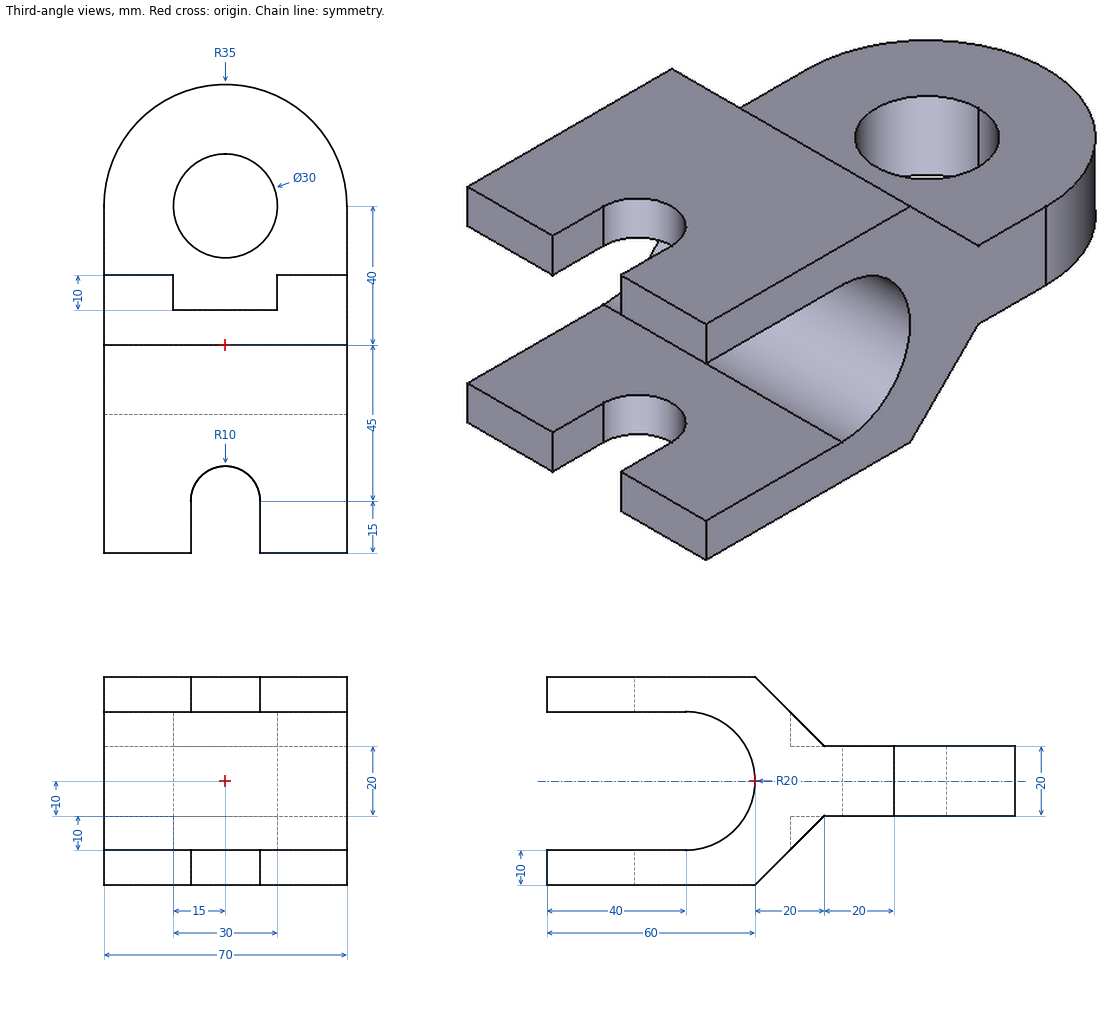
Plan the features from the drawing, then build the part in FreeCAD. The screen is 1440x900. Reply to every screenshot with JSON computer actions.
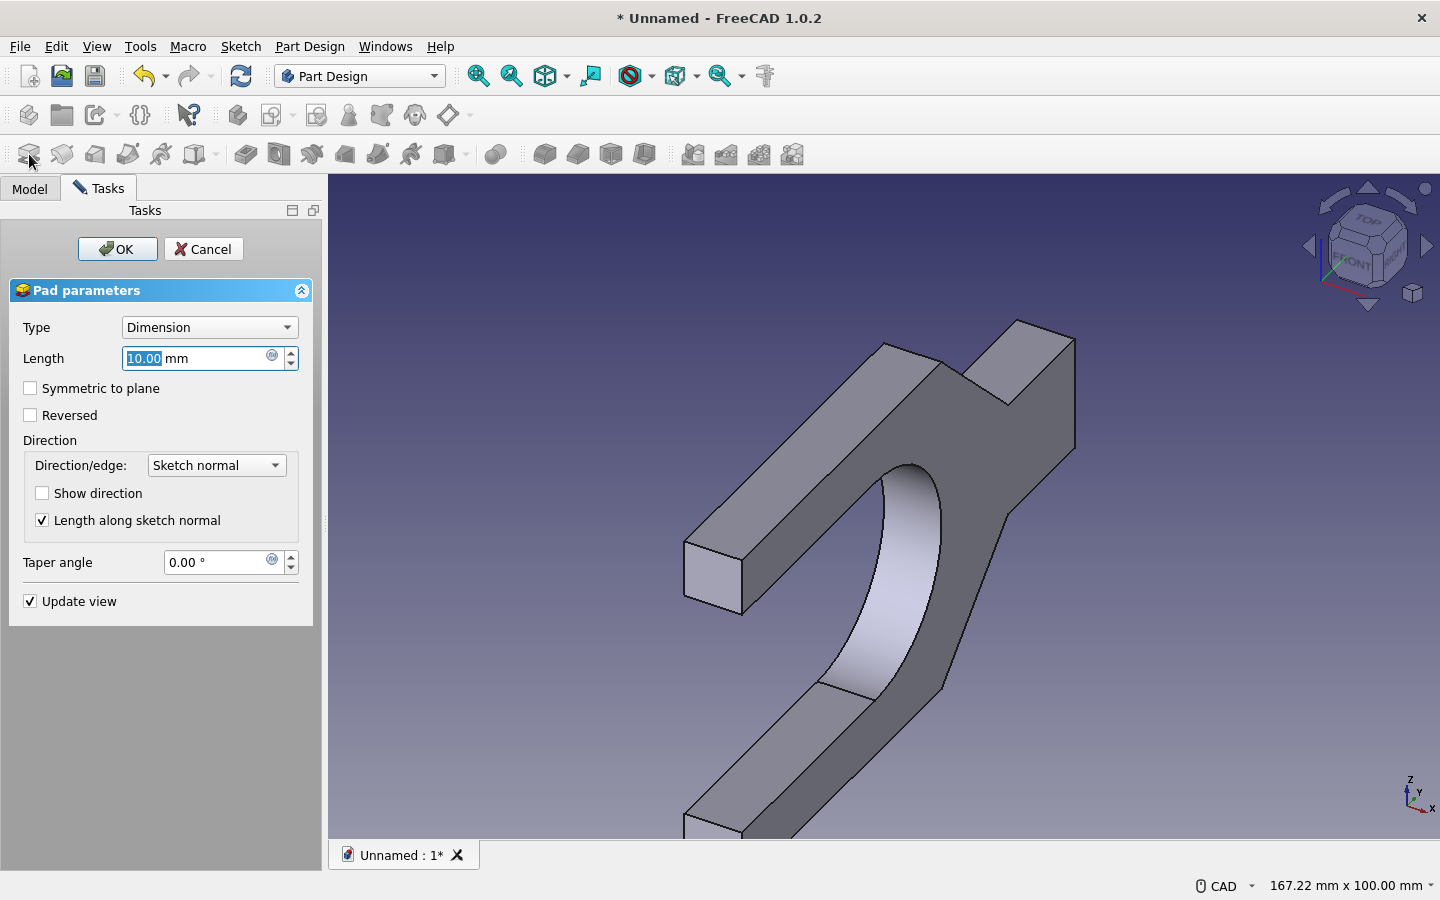
{"action": "type", "text": "70"}
{"action": "key", "text": "Tab"}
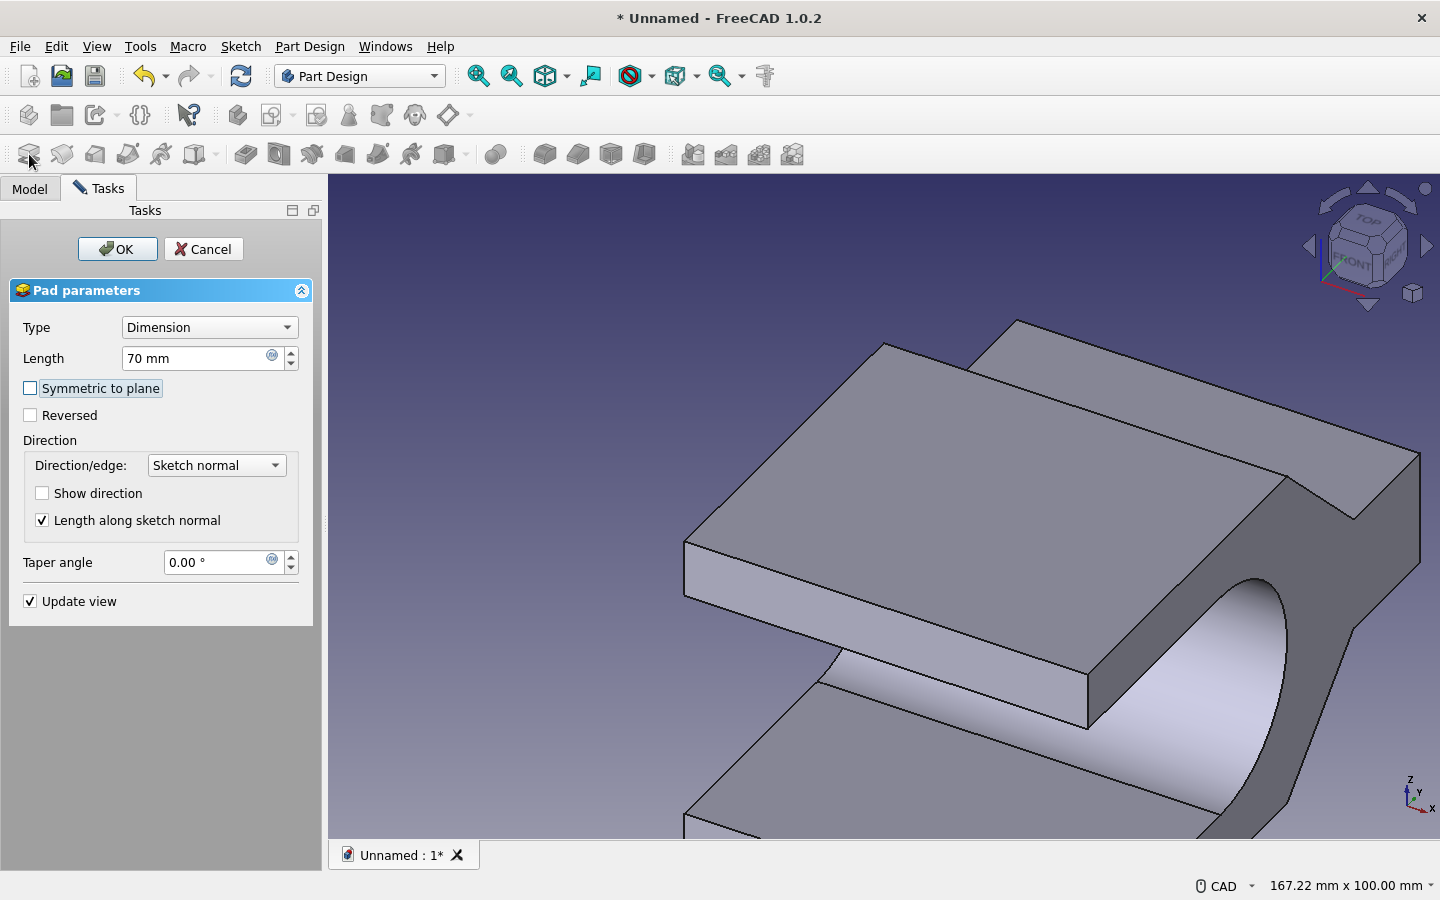
{"action": "left_click", "coordinate": [31, 388]}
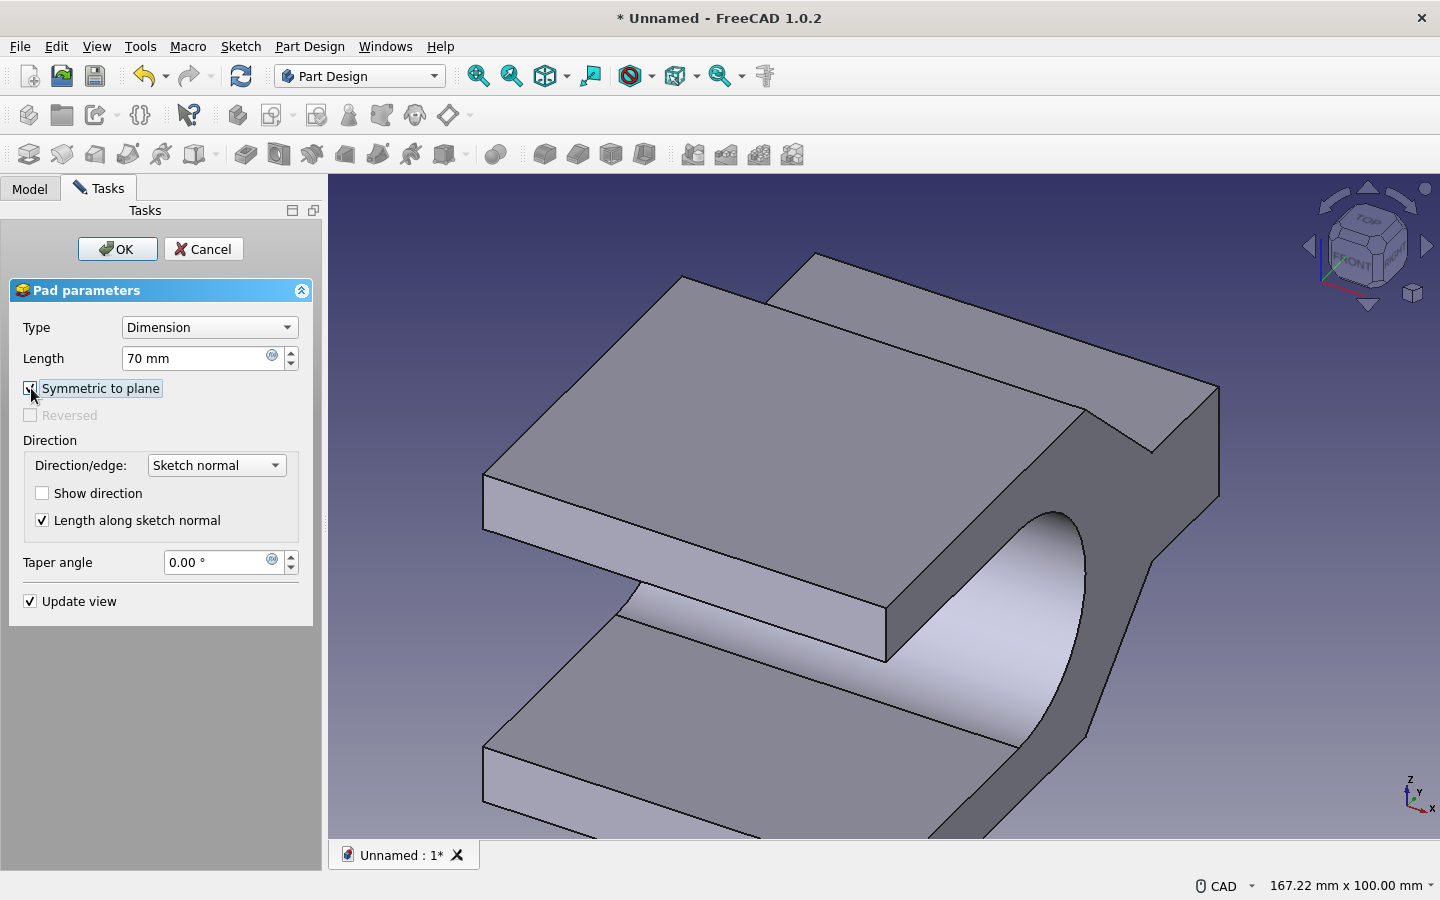
{"action": "left_click", "coordinate": [118, 249]}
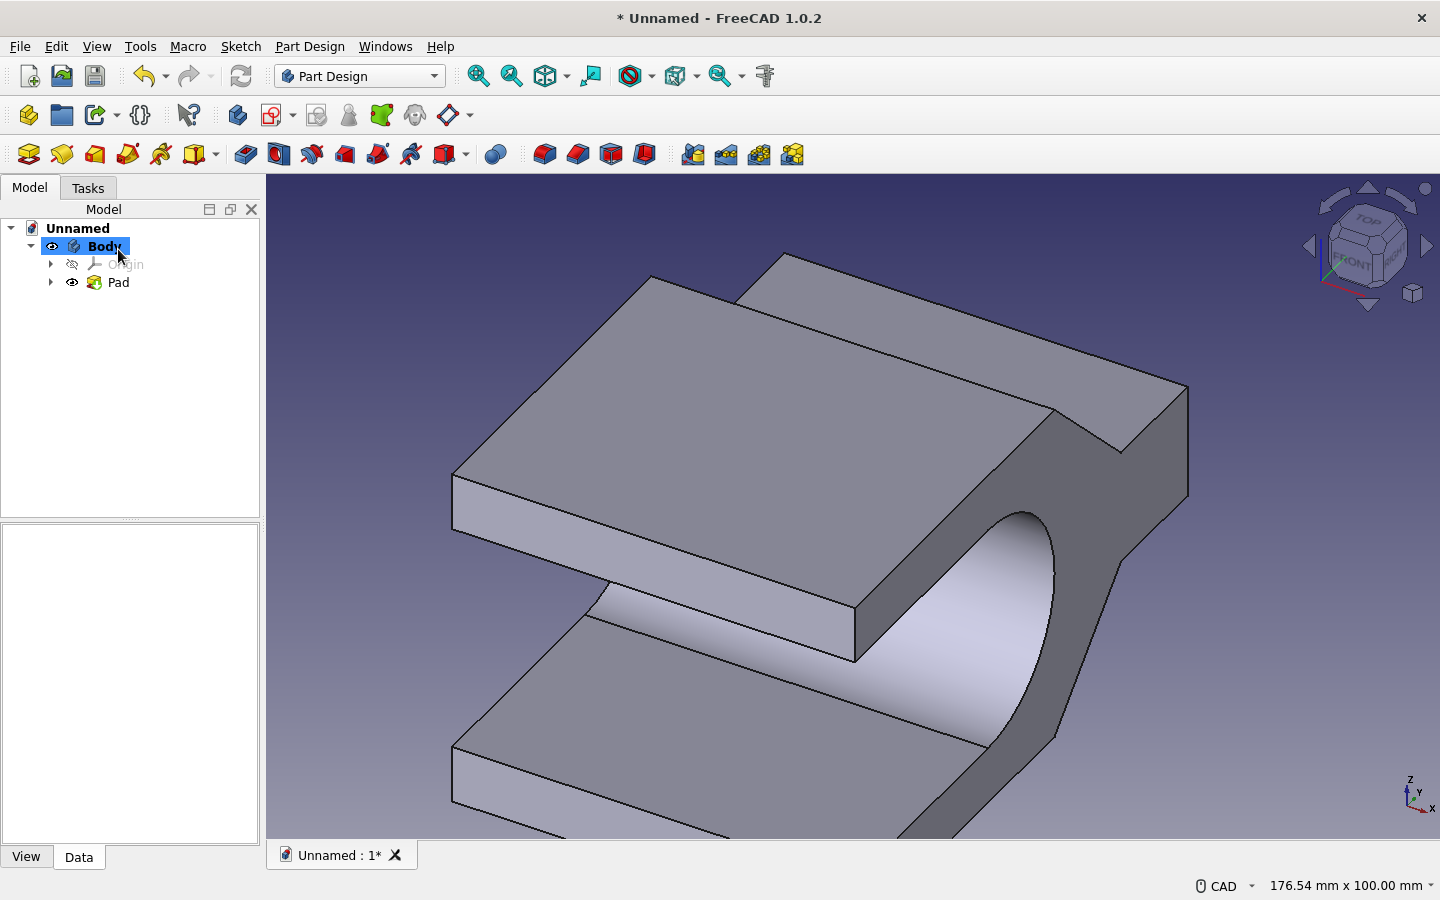
{"action": "left_click", "coordinate": [479, 76]}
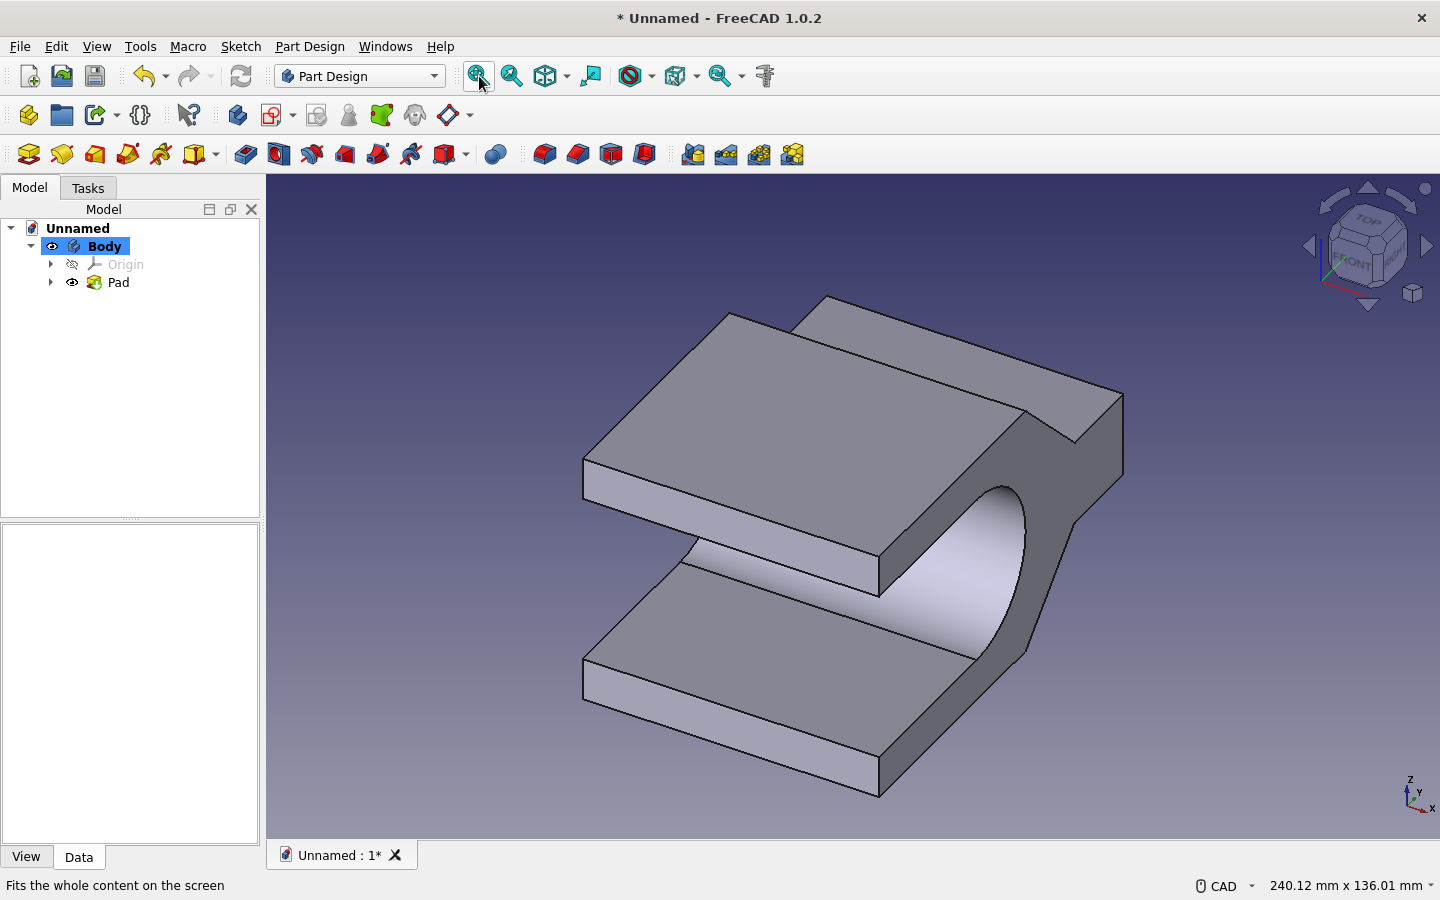
{"action": "key", "text": "5"}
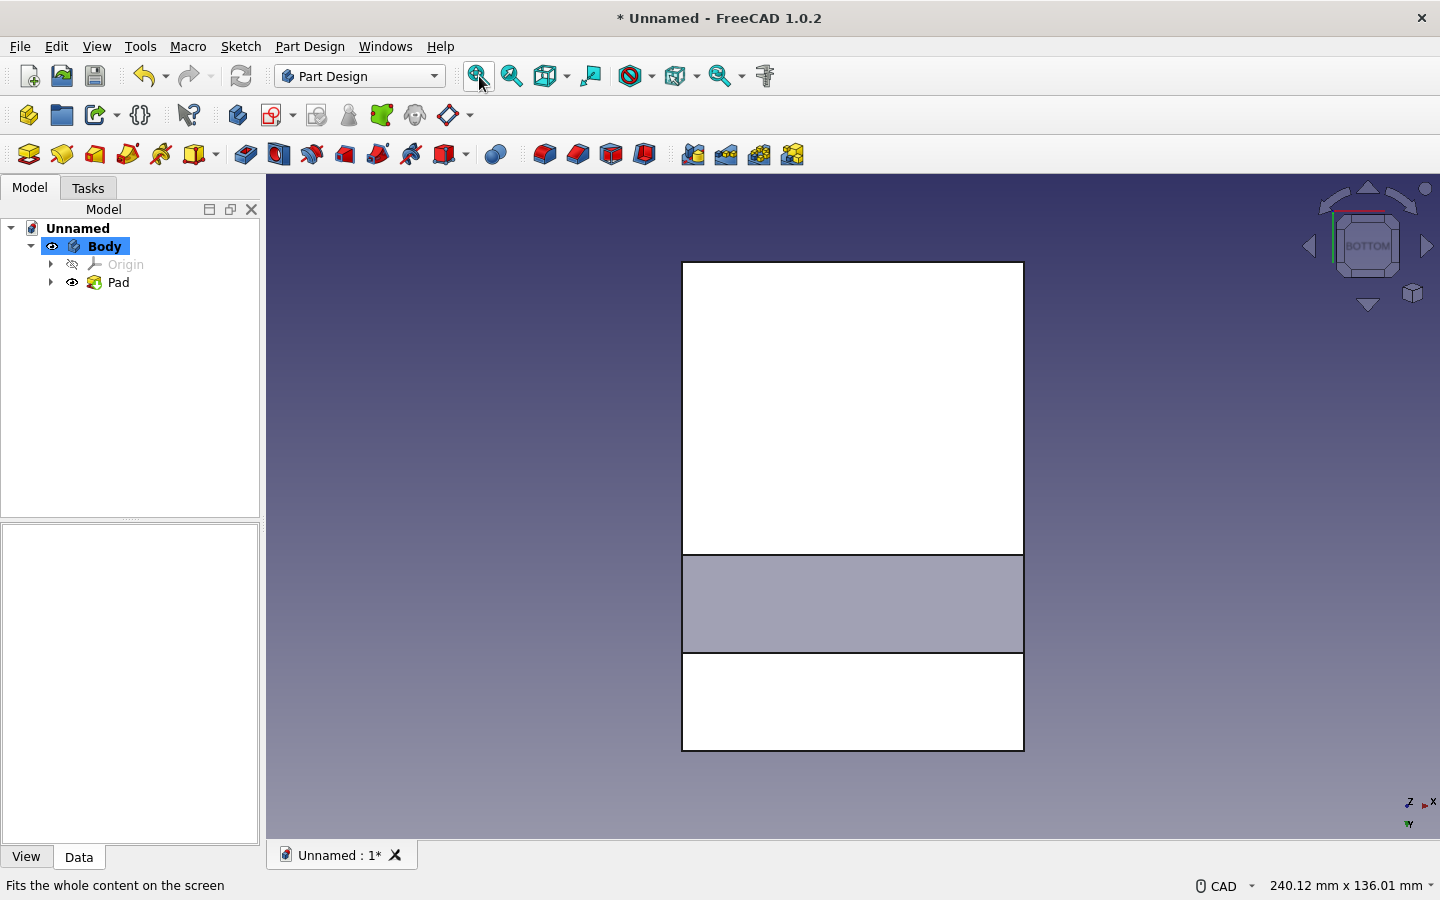
{"action": "left_click", "coordinate": [902, 701]}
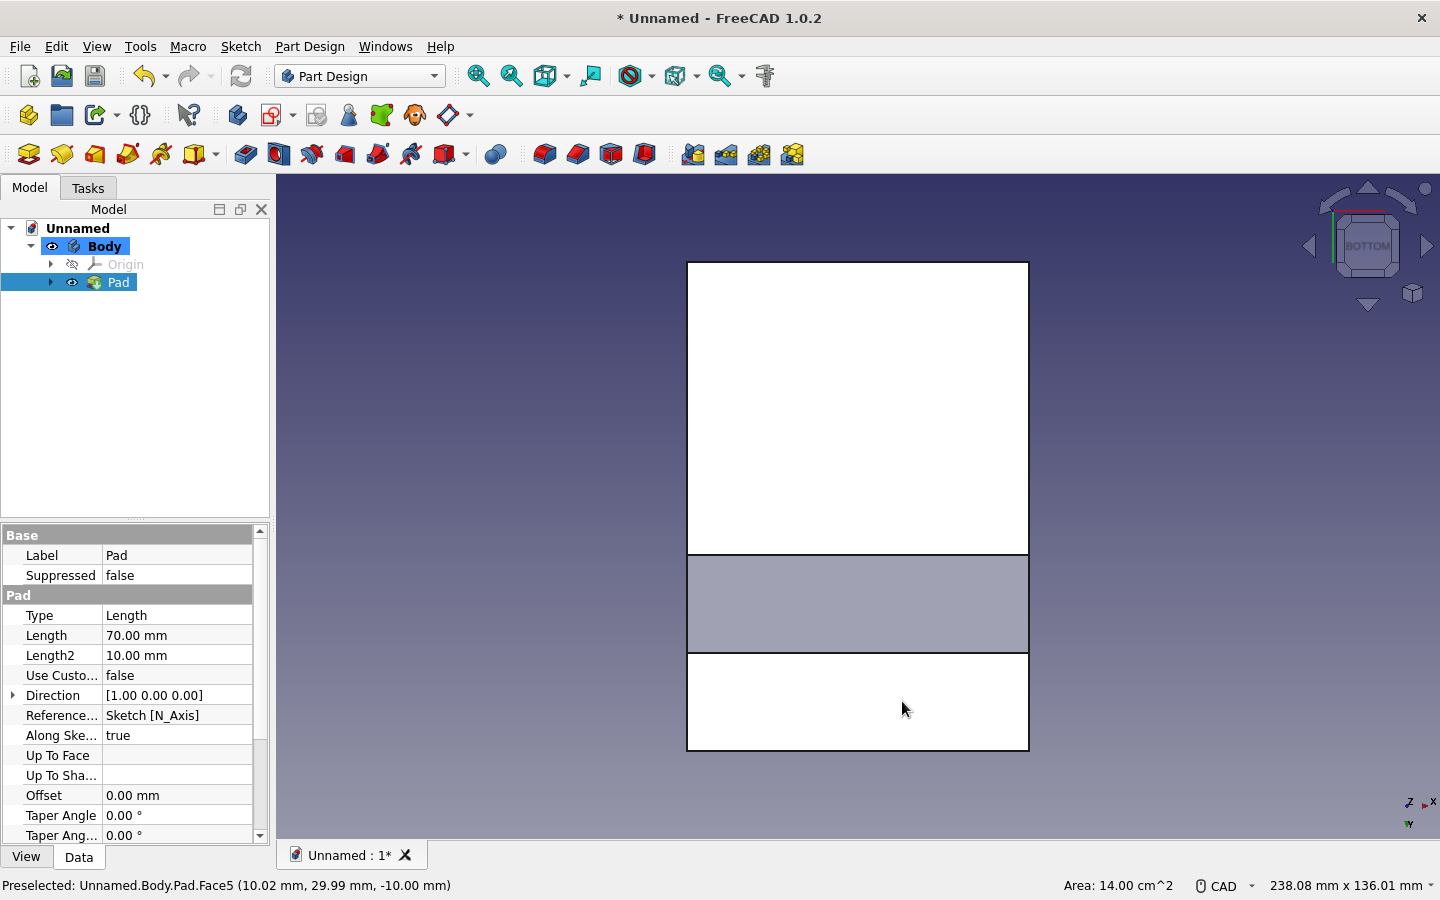
{"action": "left_click", "coordinate": [270, 116]}